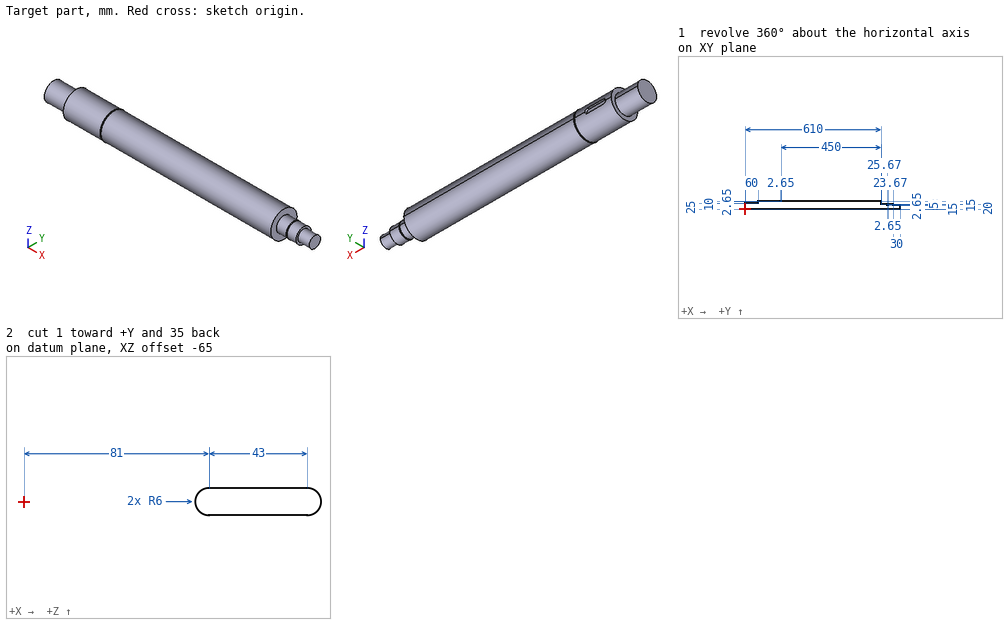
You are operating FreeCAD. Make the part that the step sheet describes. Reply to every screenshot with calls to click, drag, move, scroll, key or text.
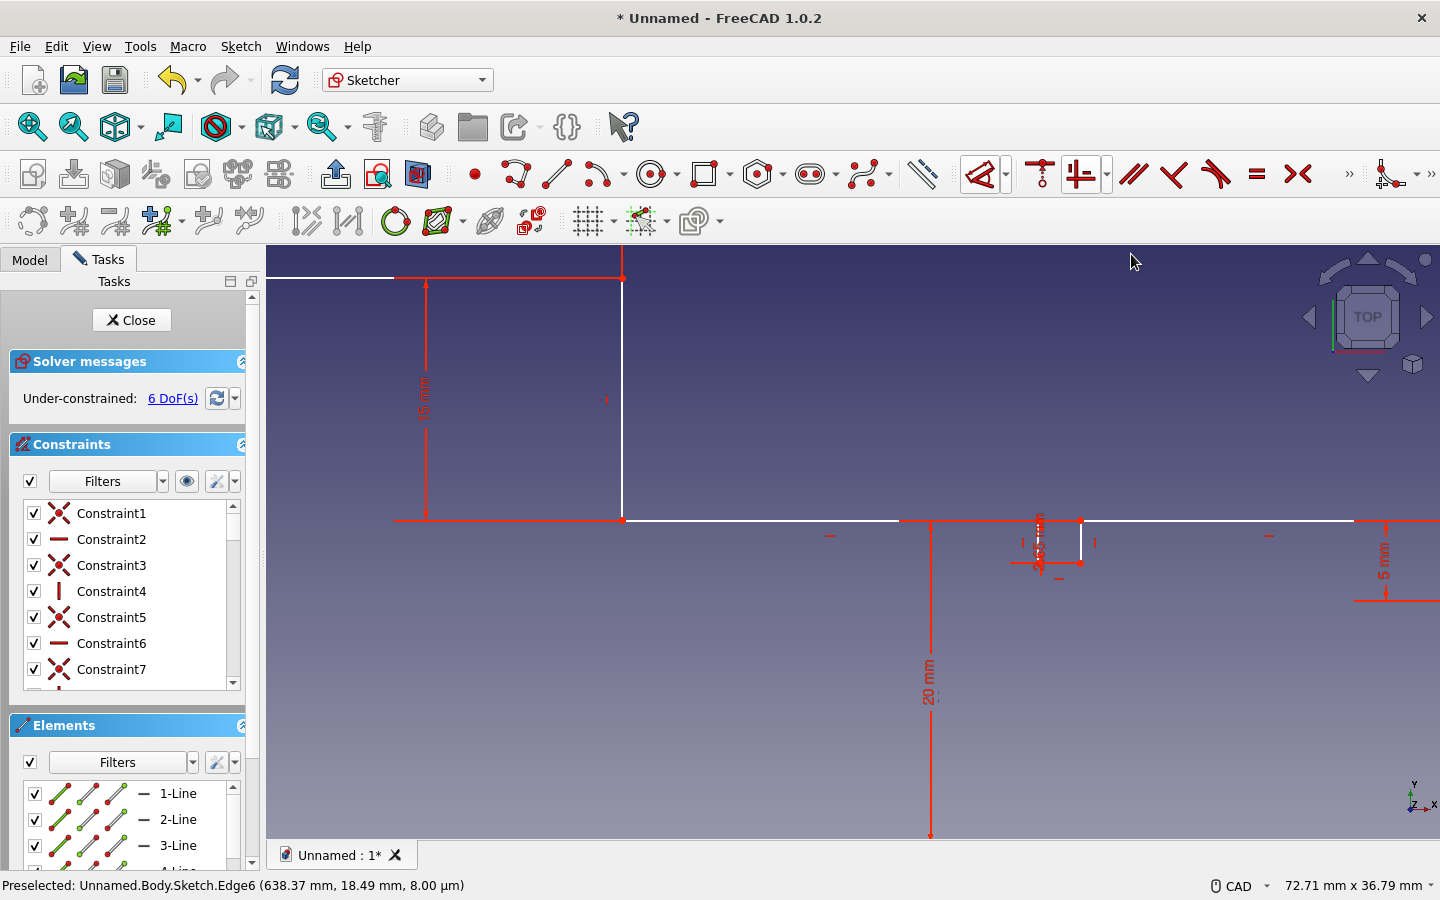
click(1068, 563)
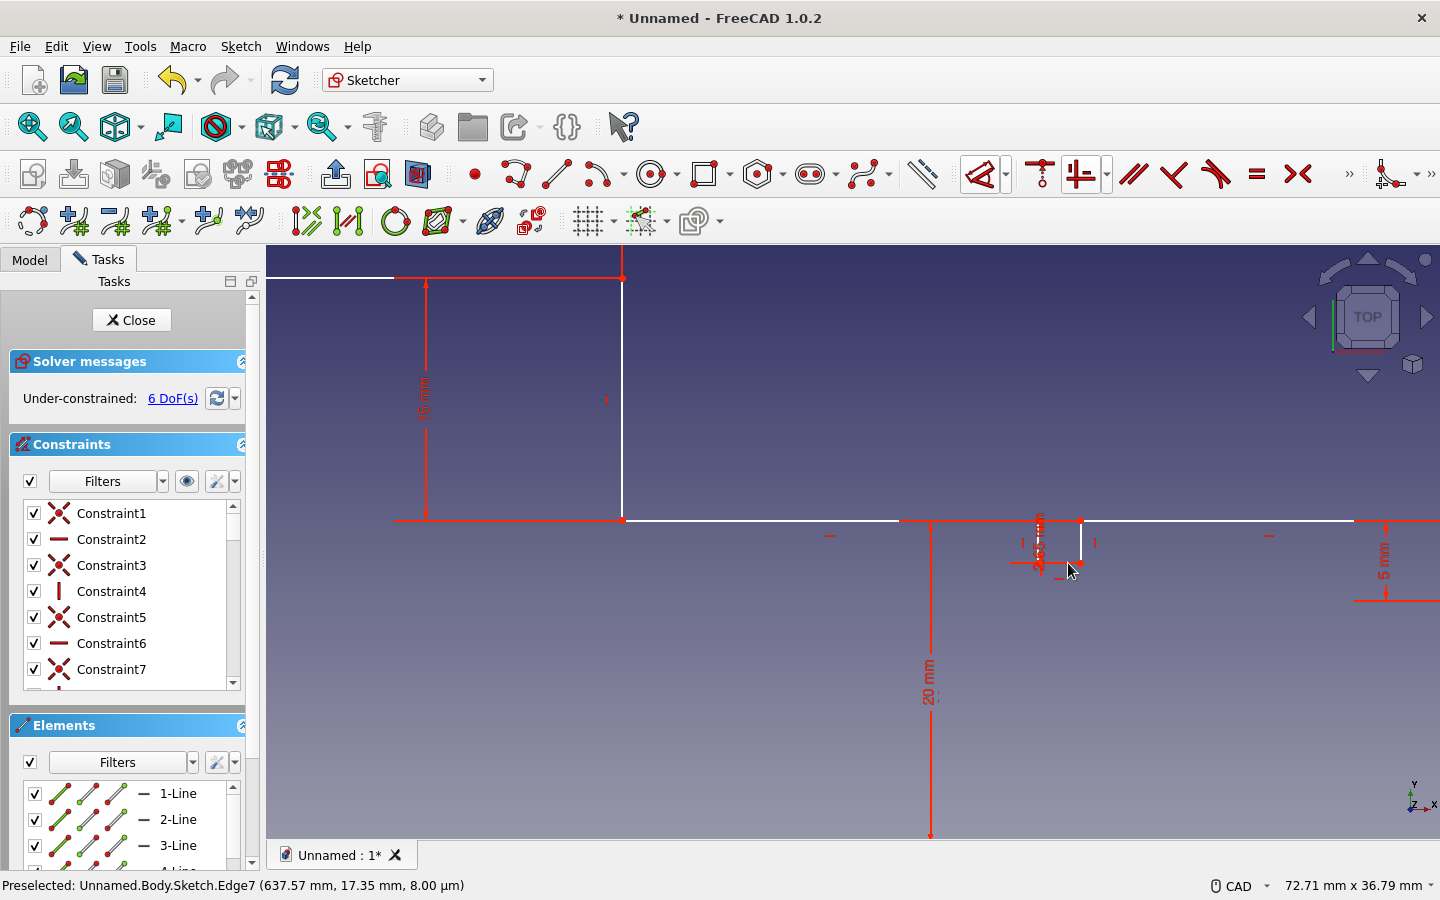
click(1006, 174)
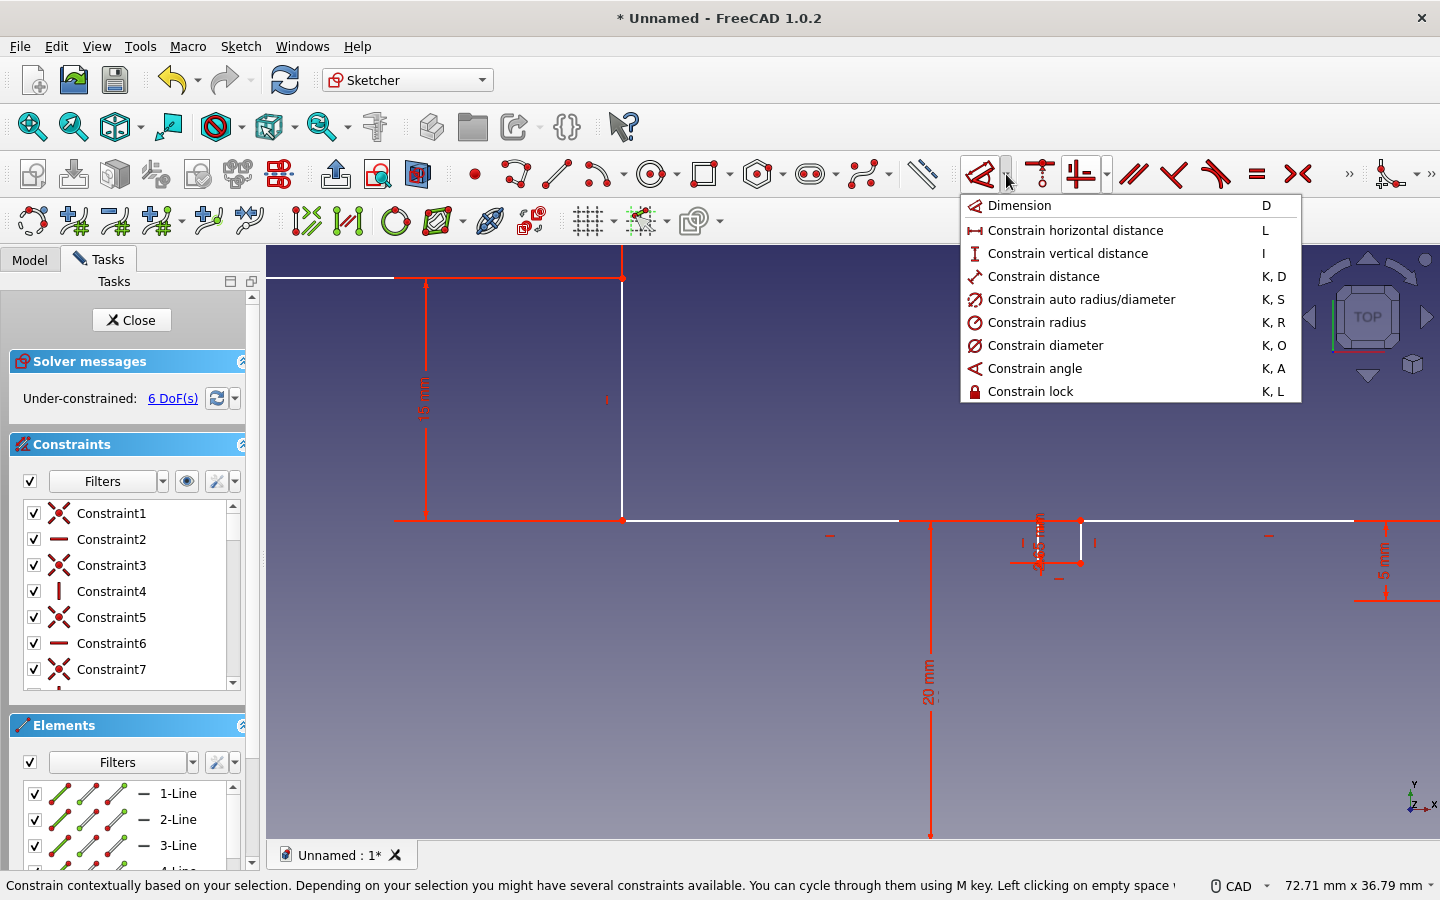
click(1131, 230)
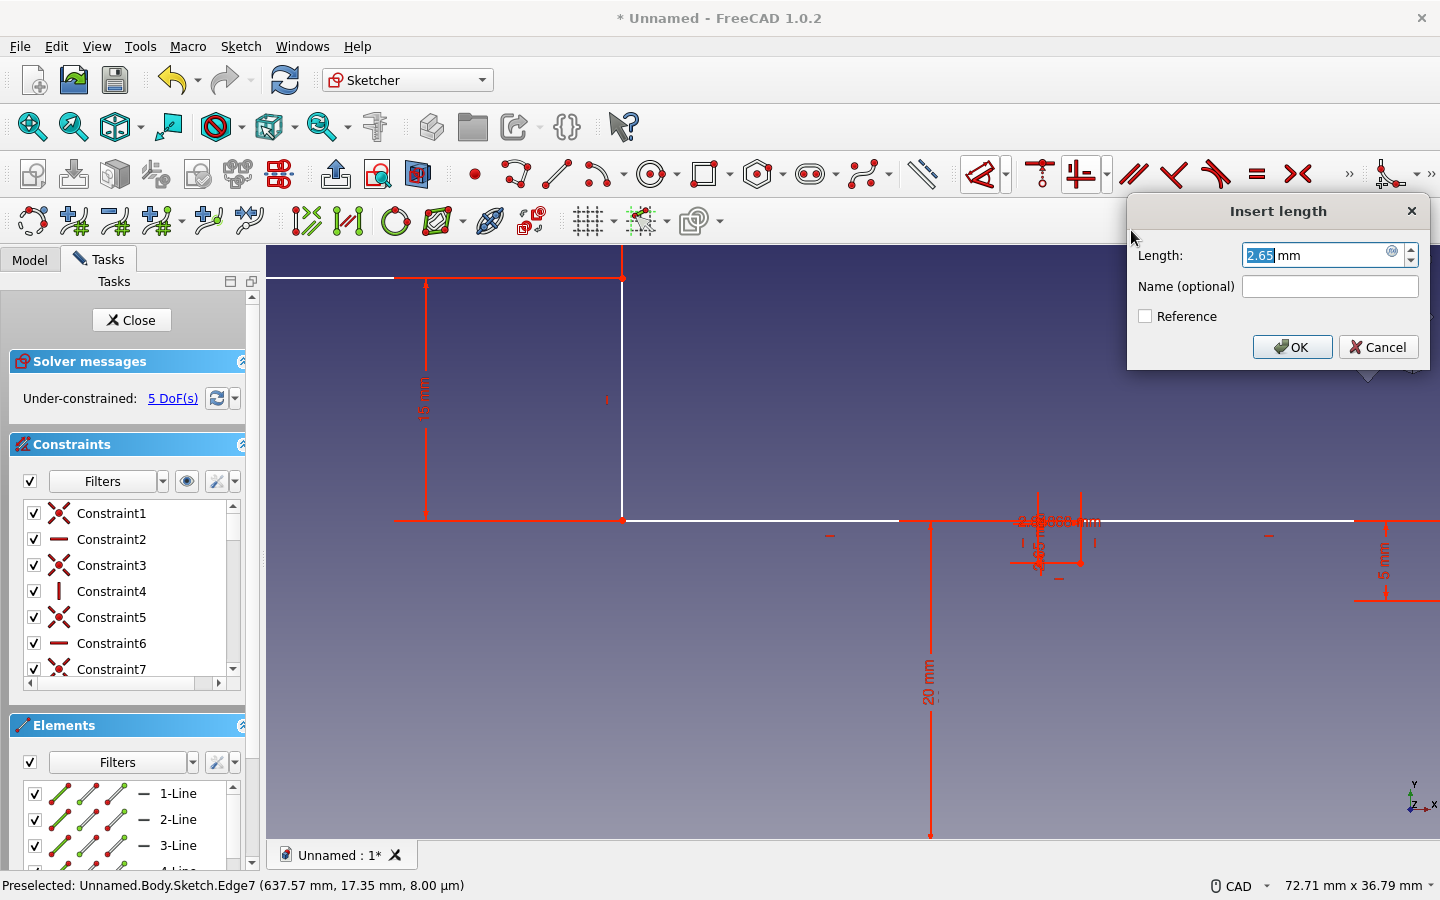
text(2.65)
key(Return)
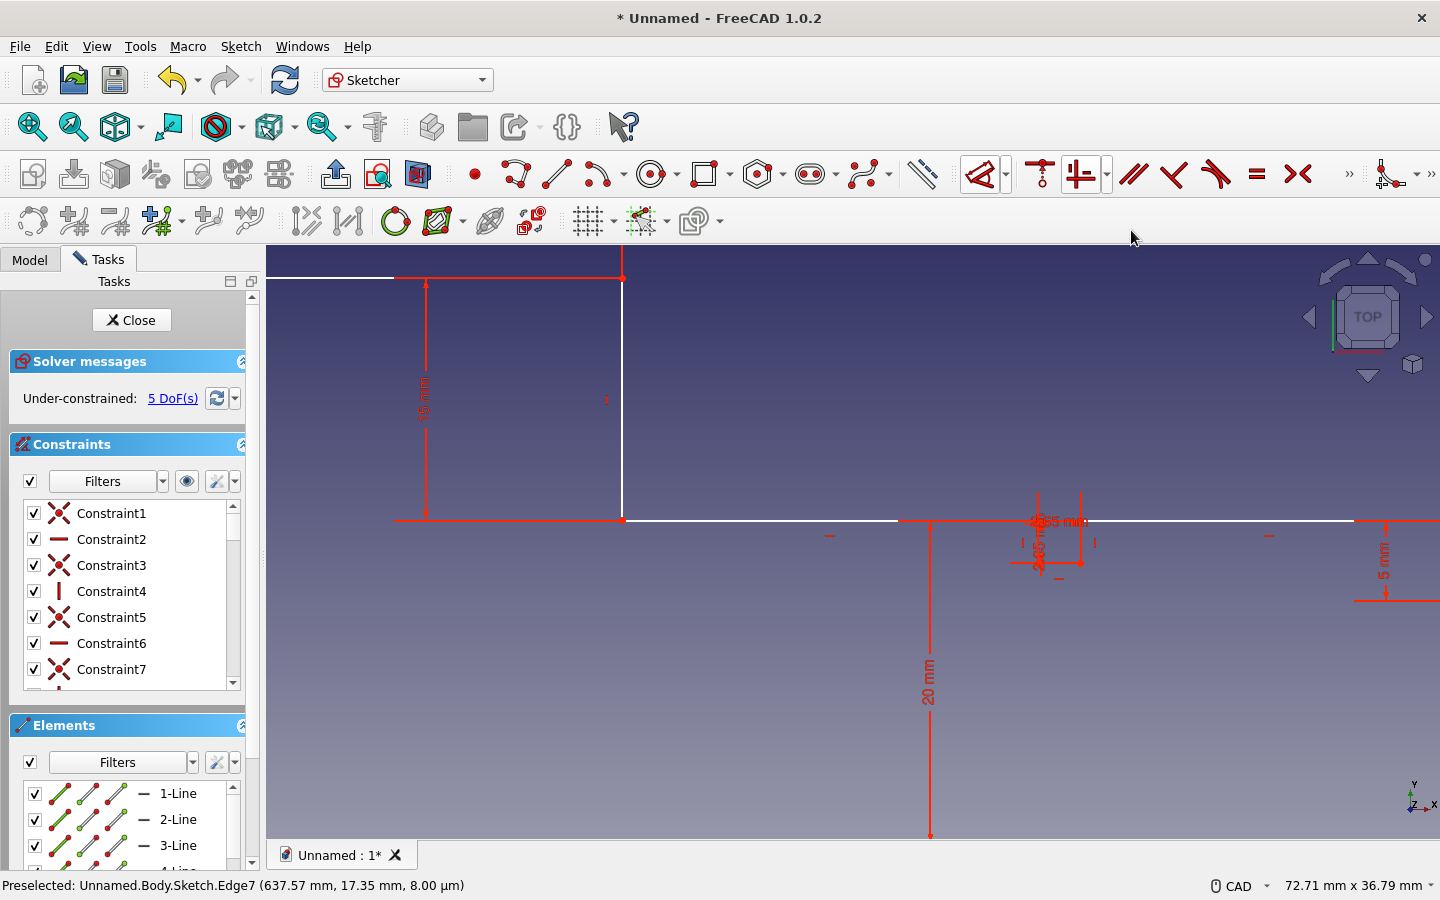
scroll(1071, 541, down, 14)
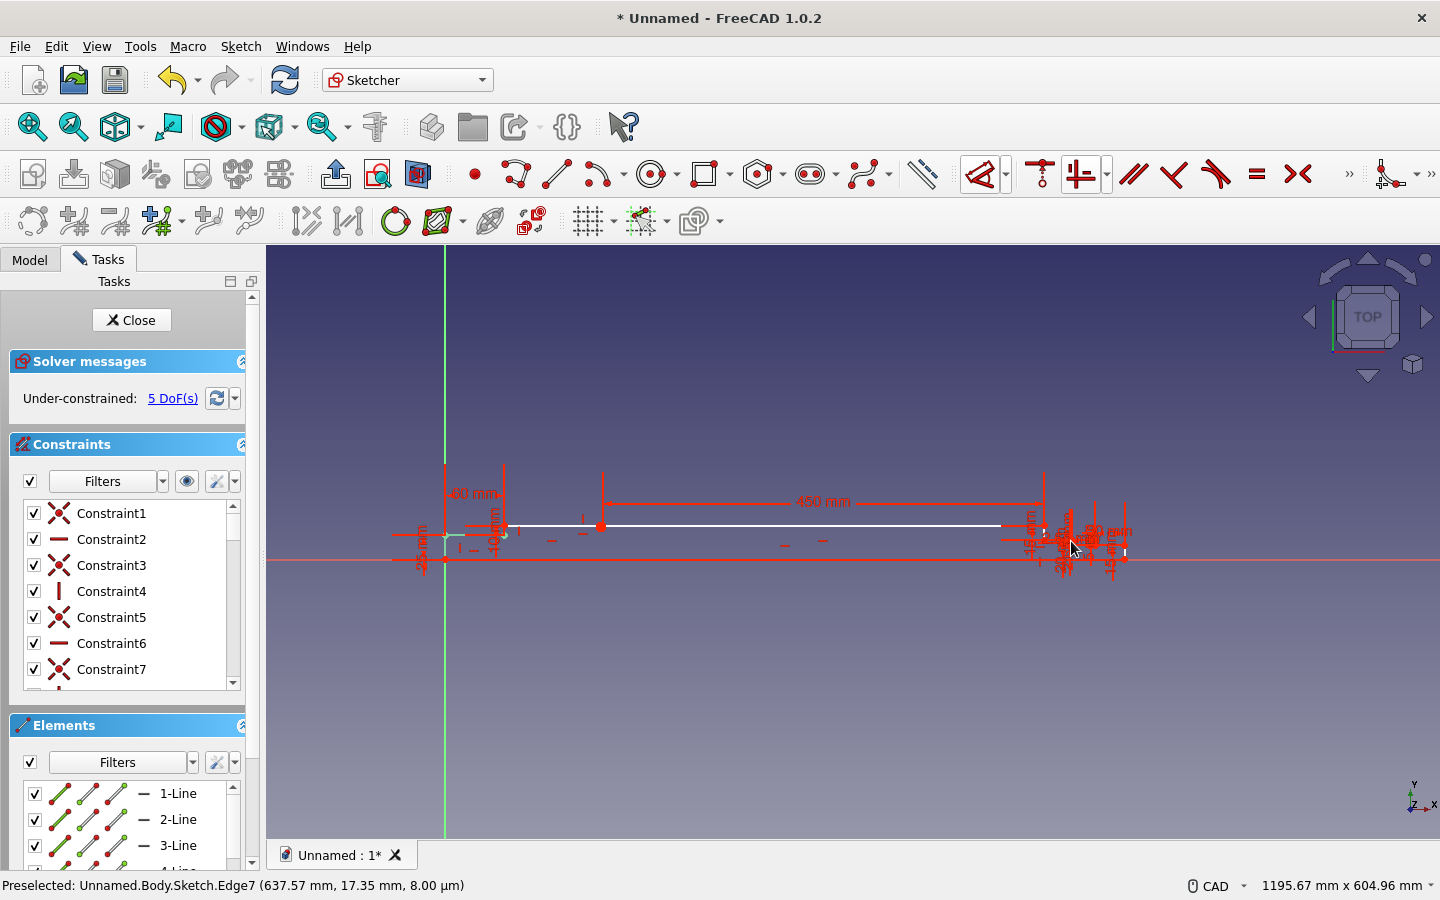
scroll(603, 526, up, 14)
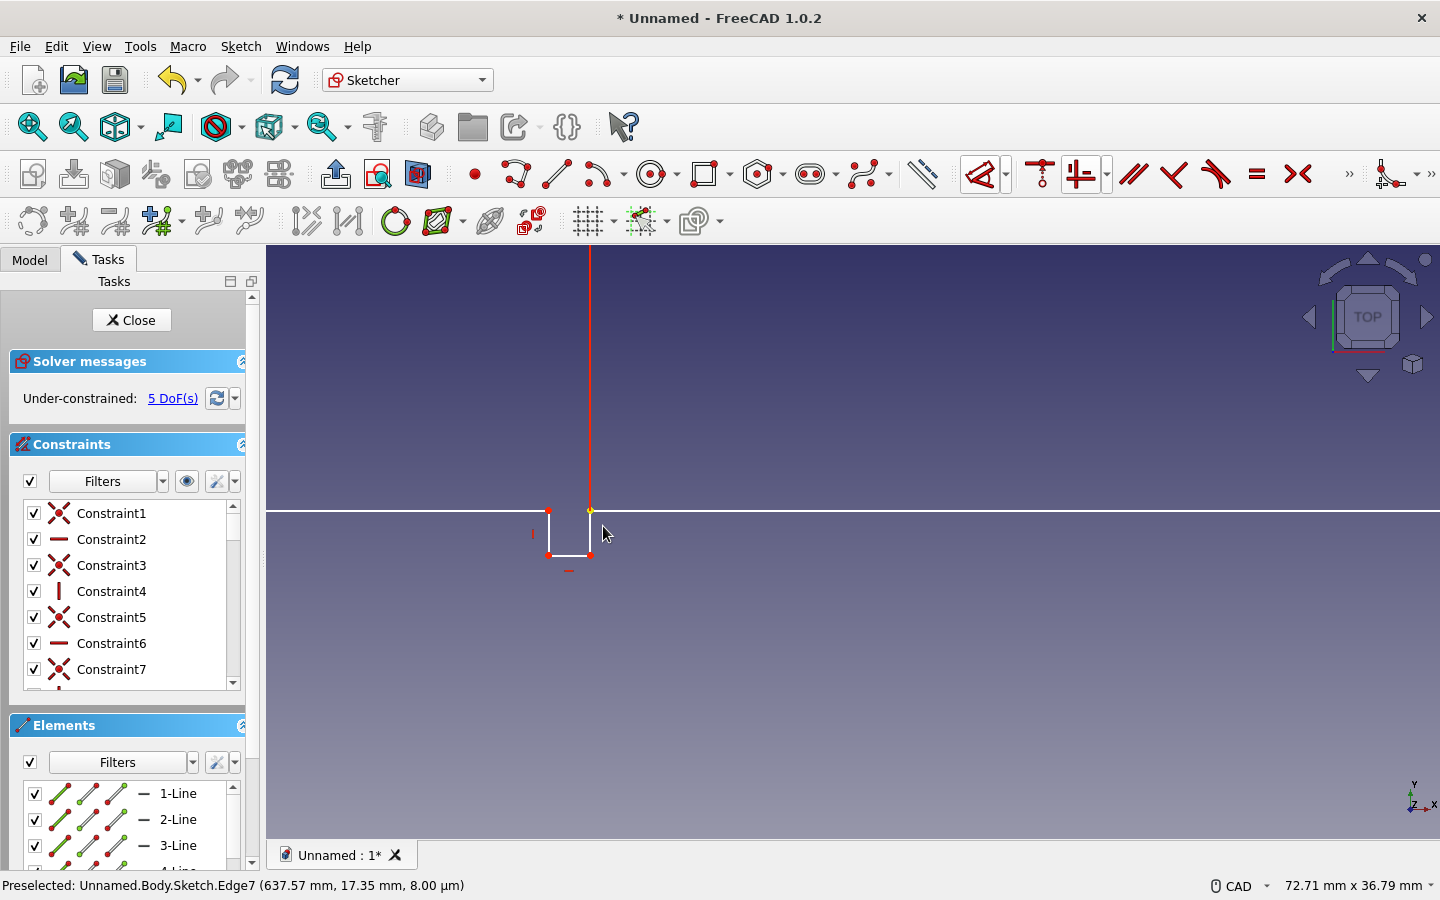
click(590, 524)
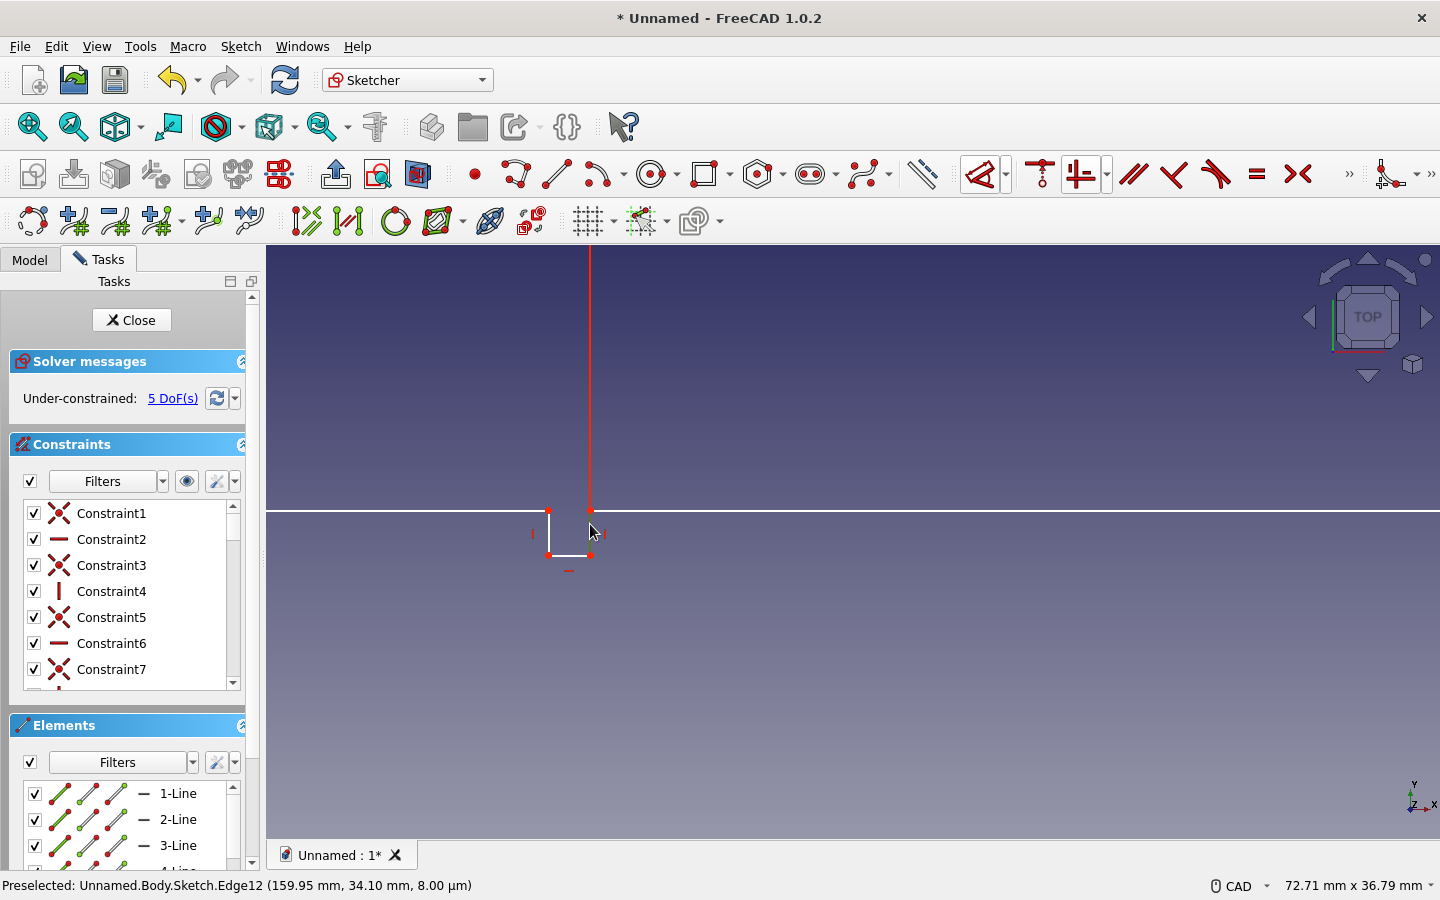
click(1006, 174)